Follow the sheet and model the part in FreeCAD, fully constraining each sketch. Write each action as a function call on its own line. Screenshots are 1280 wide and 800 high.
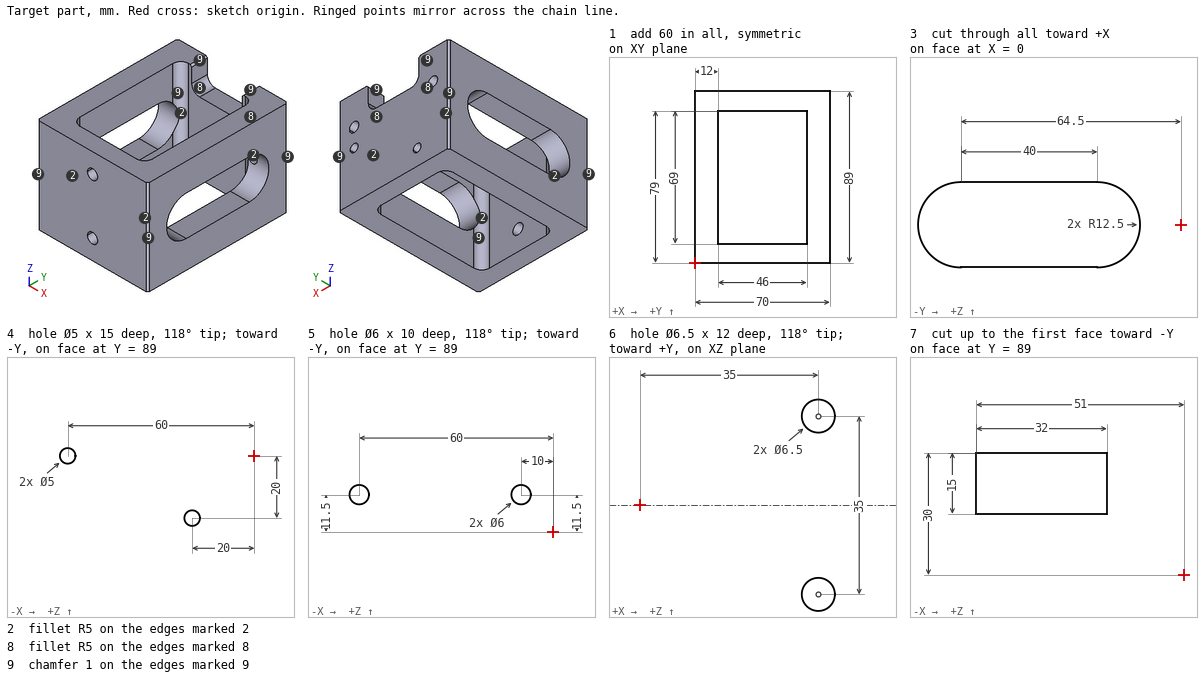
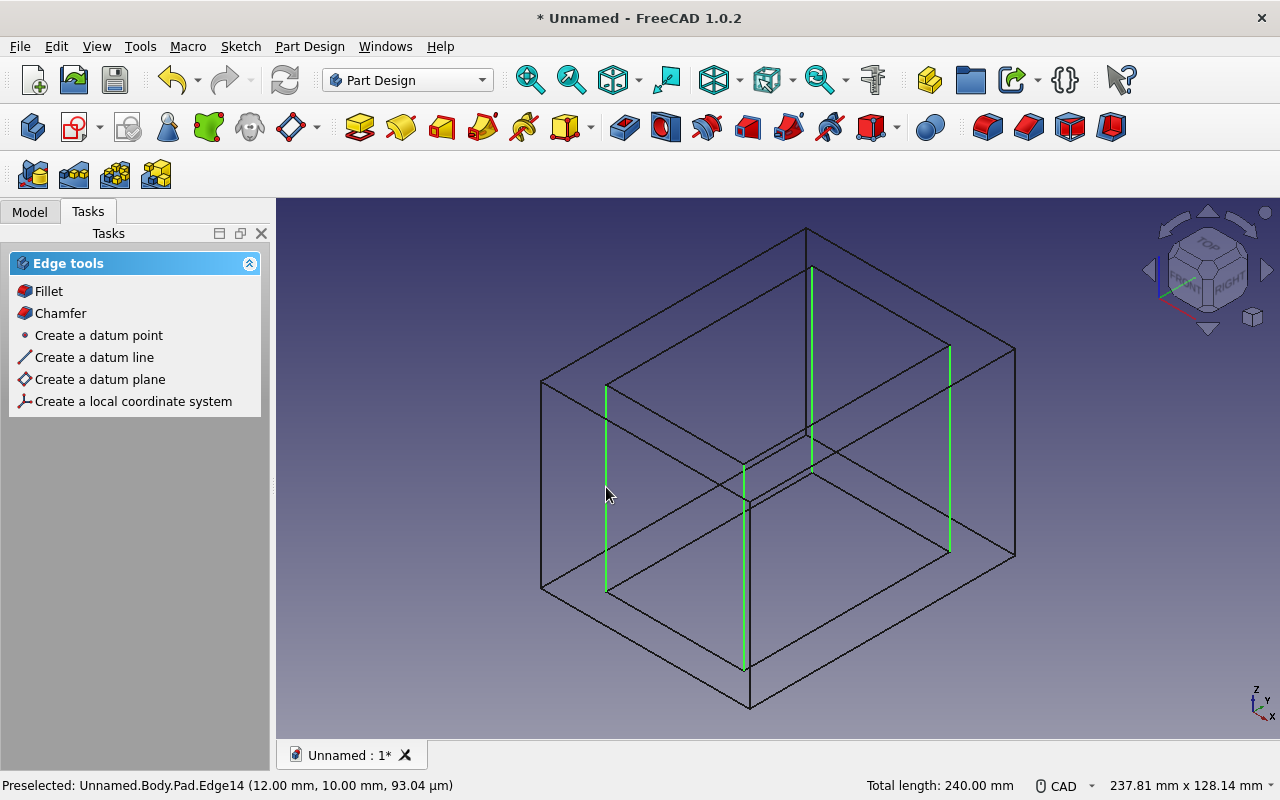
key(v)
key(1)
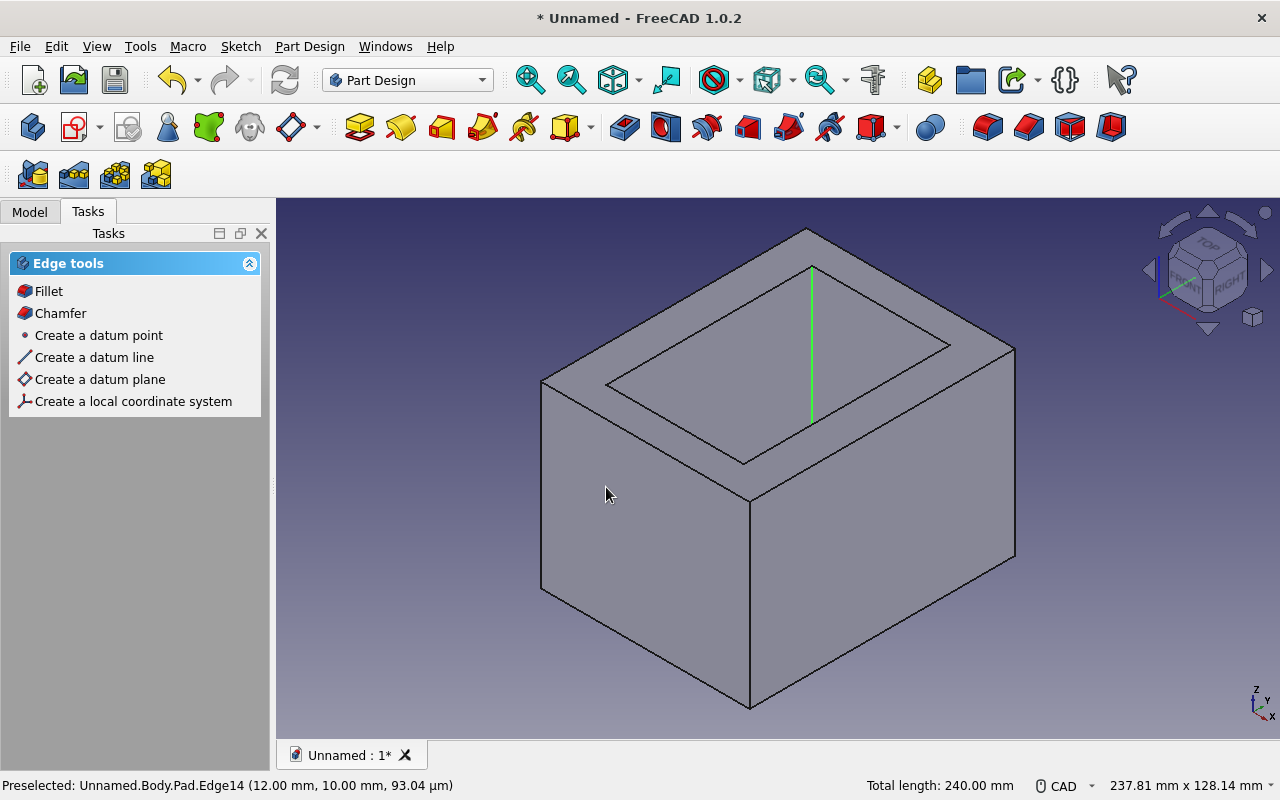
click(988, 128)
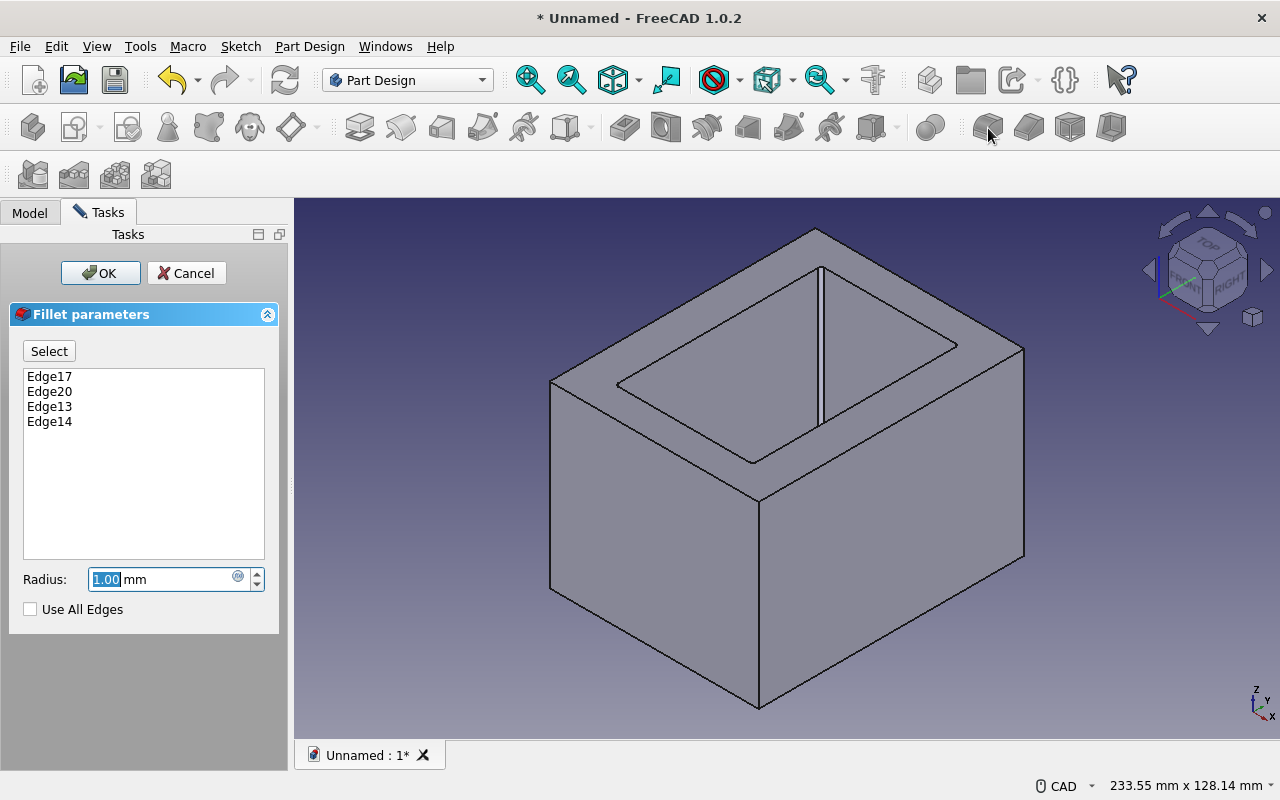
text(5)
key(Tab)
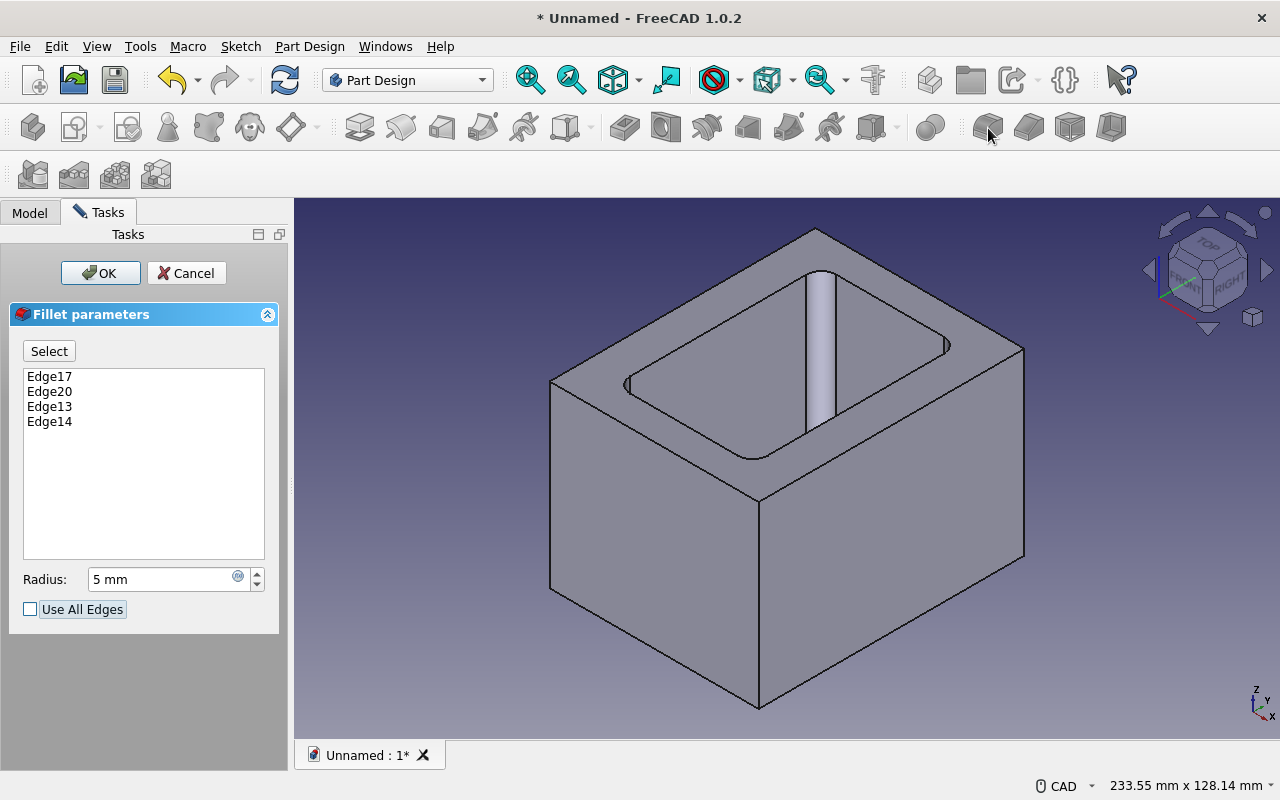
click(101, 273)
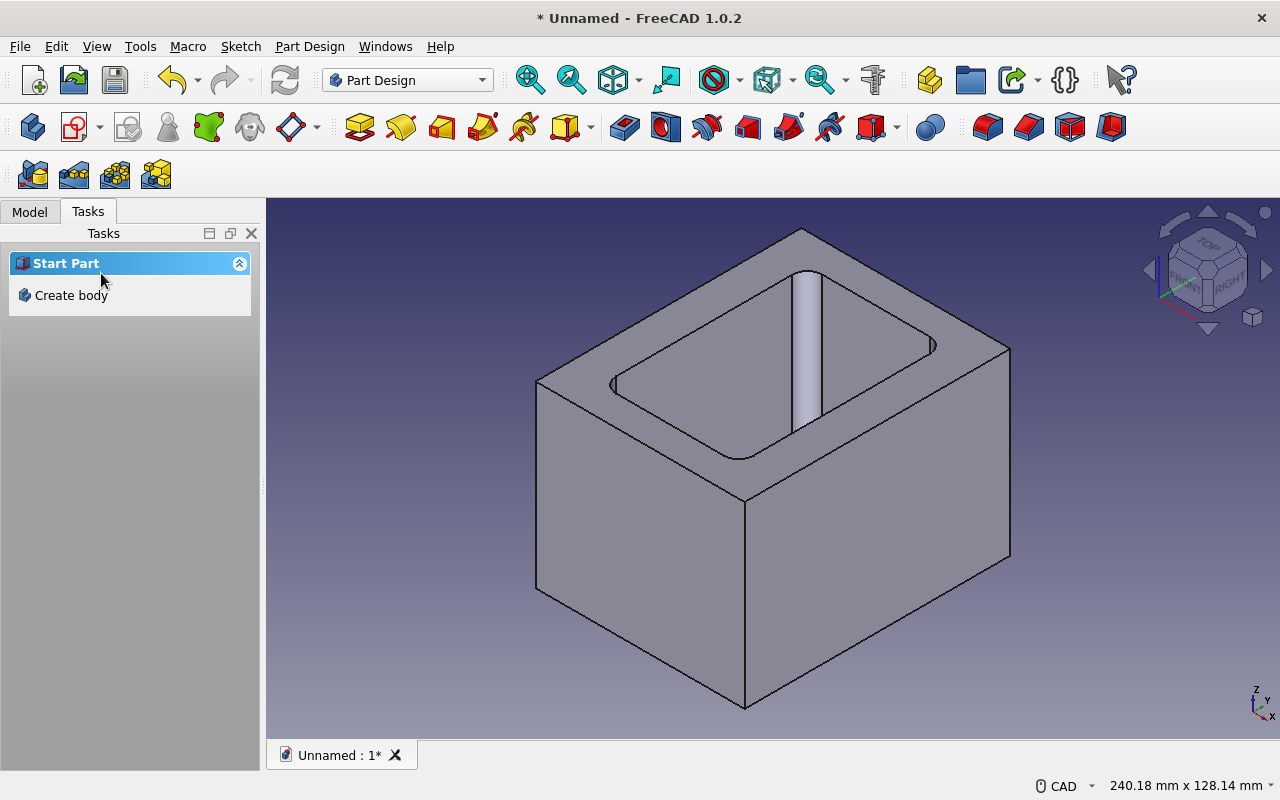
key(6)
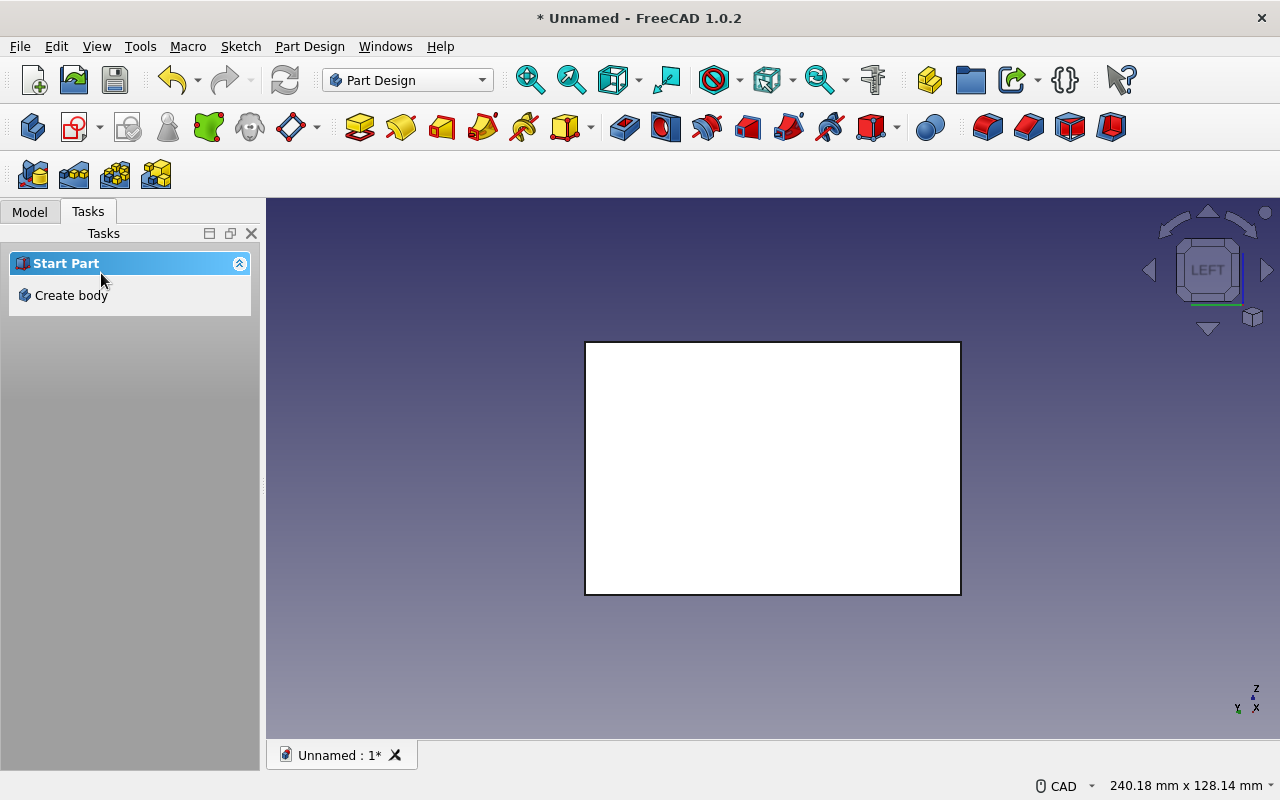
click(719, 467)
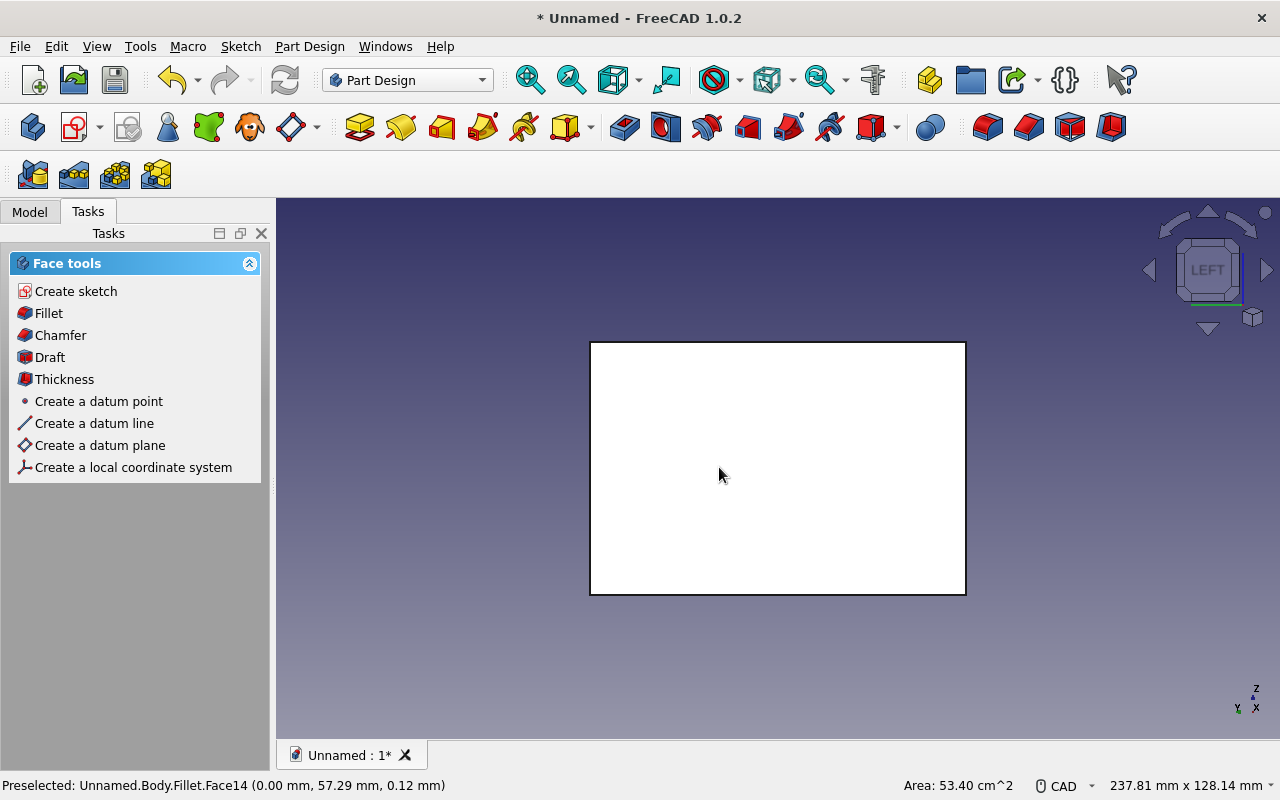
click(74, 128)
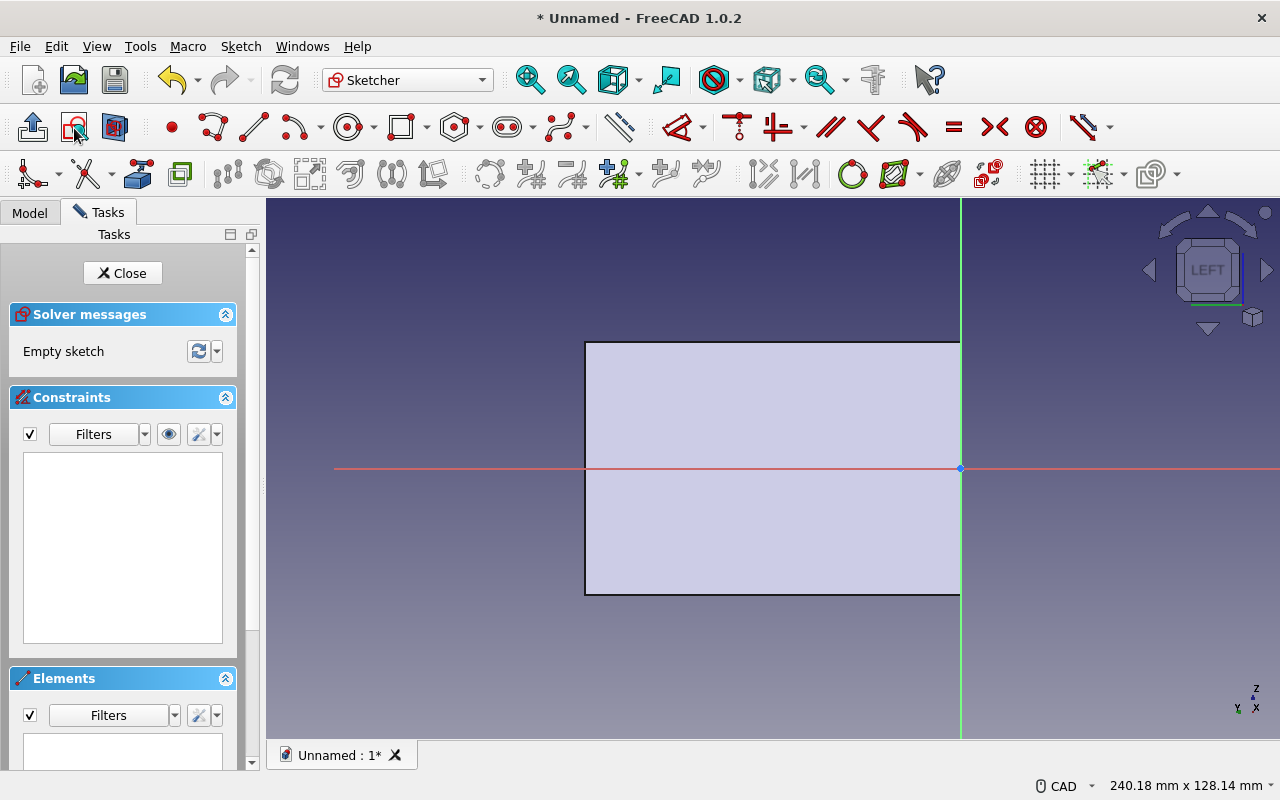
scroll(912, 468, up, 3)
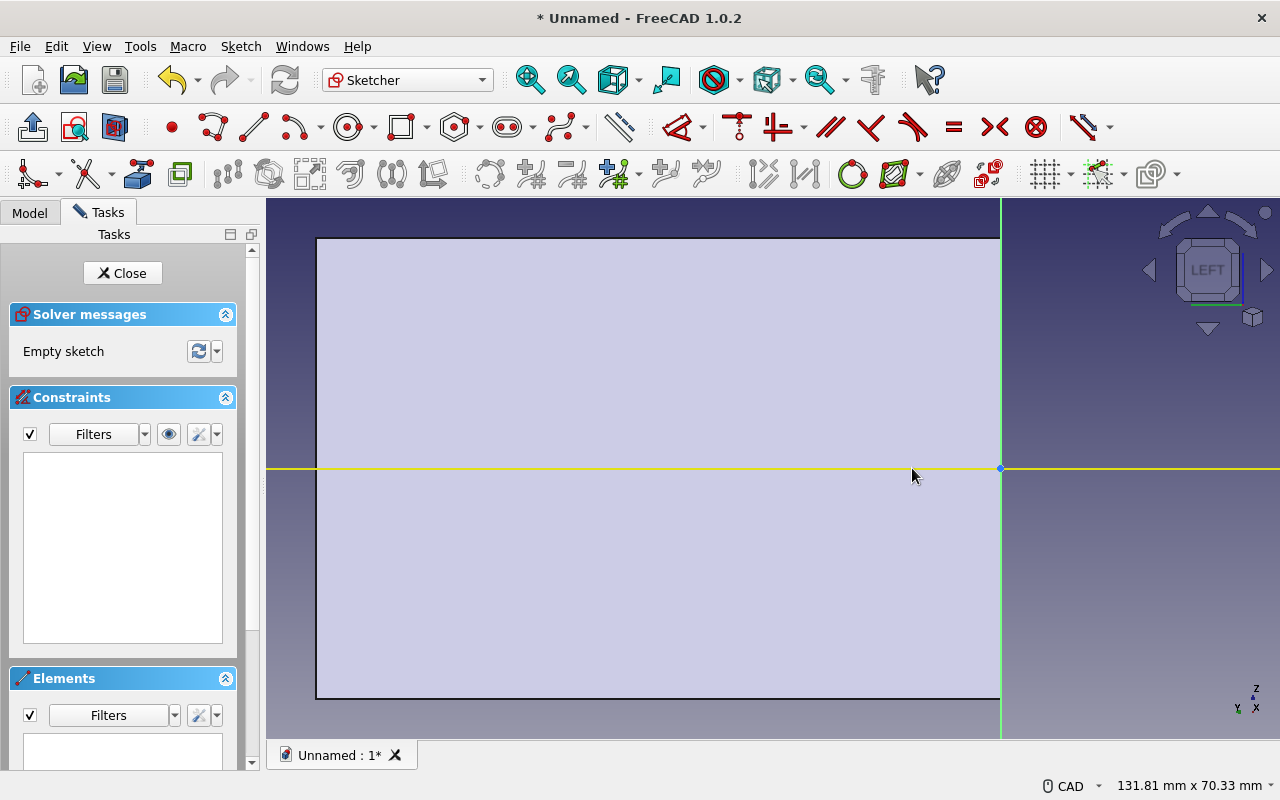
click(506, 128)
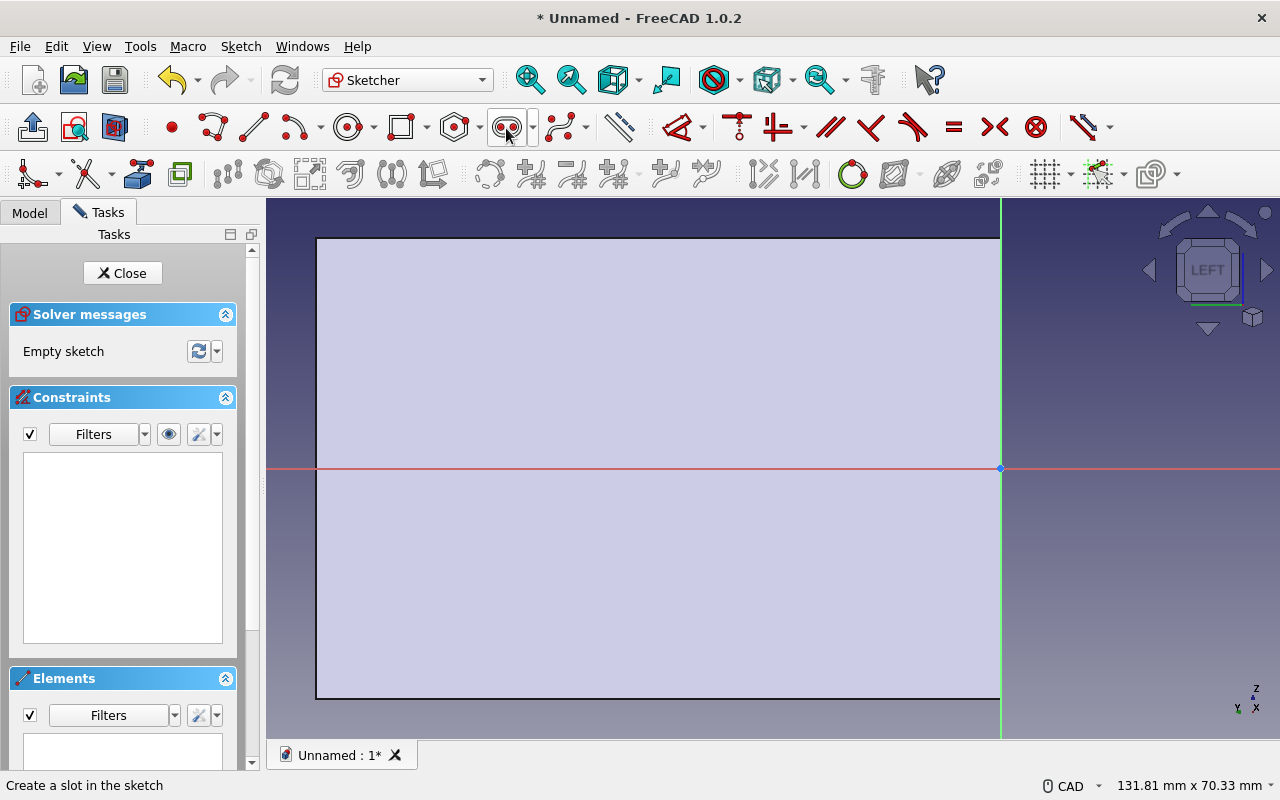
click(504, 468)